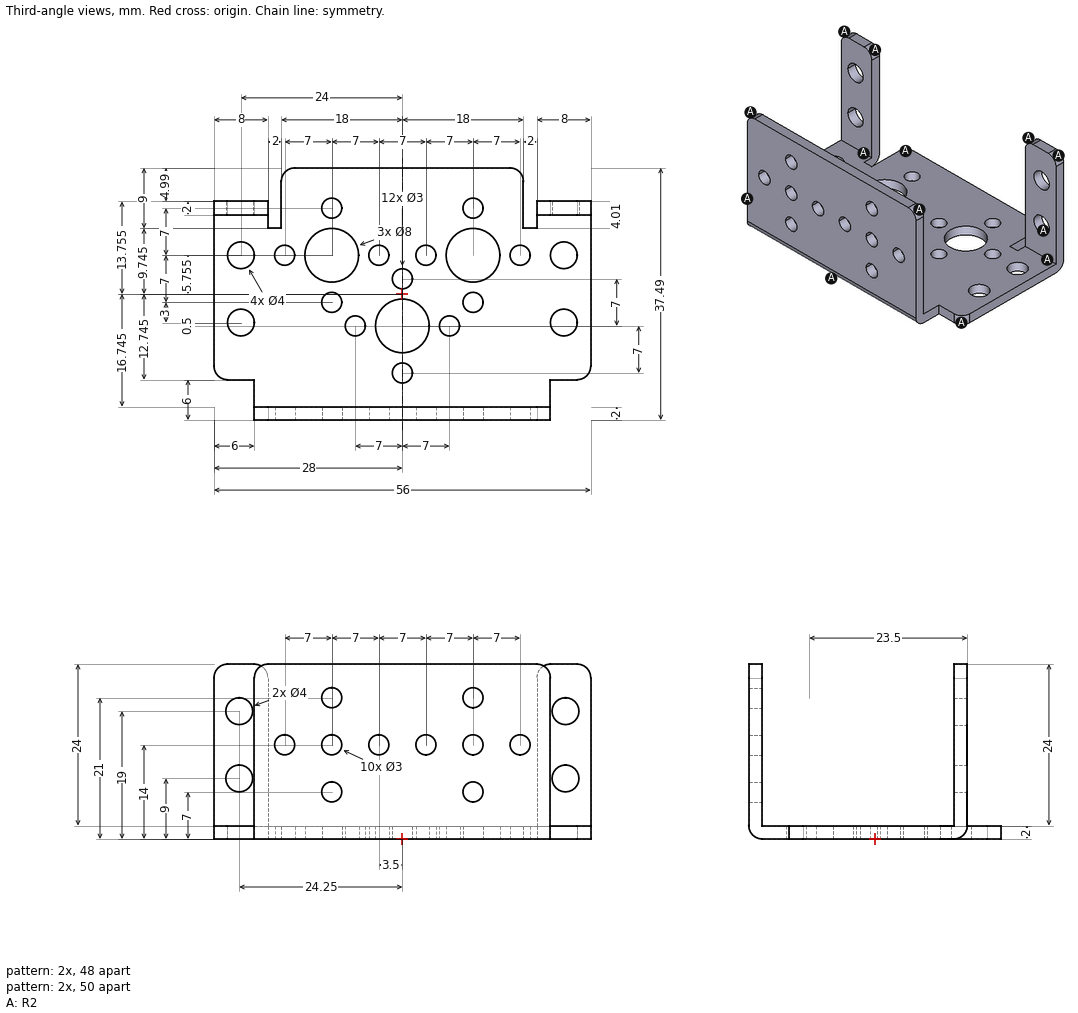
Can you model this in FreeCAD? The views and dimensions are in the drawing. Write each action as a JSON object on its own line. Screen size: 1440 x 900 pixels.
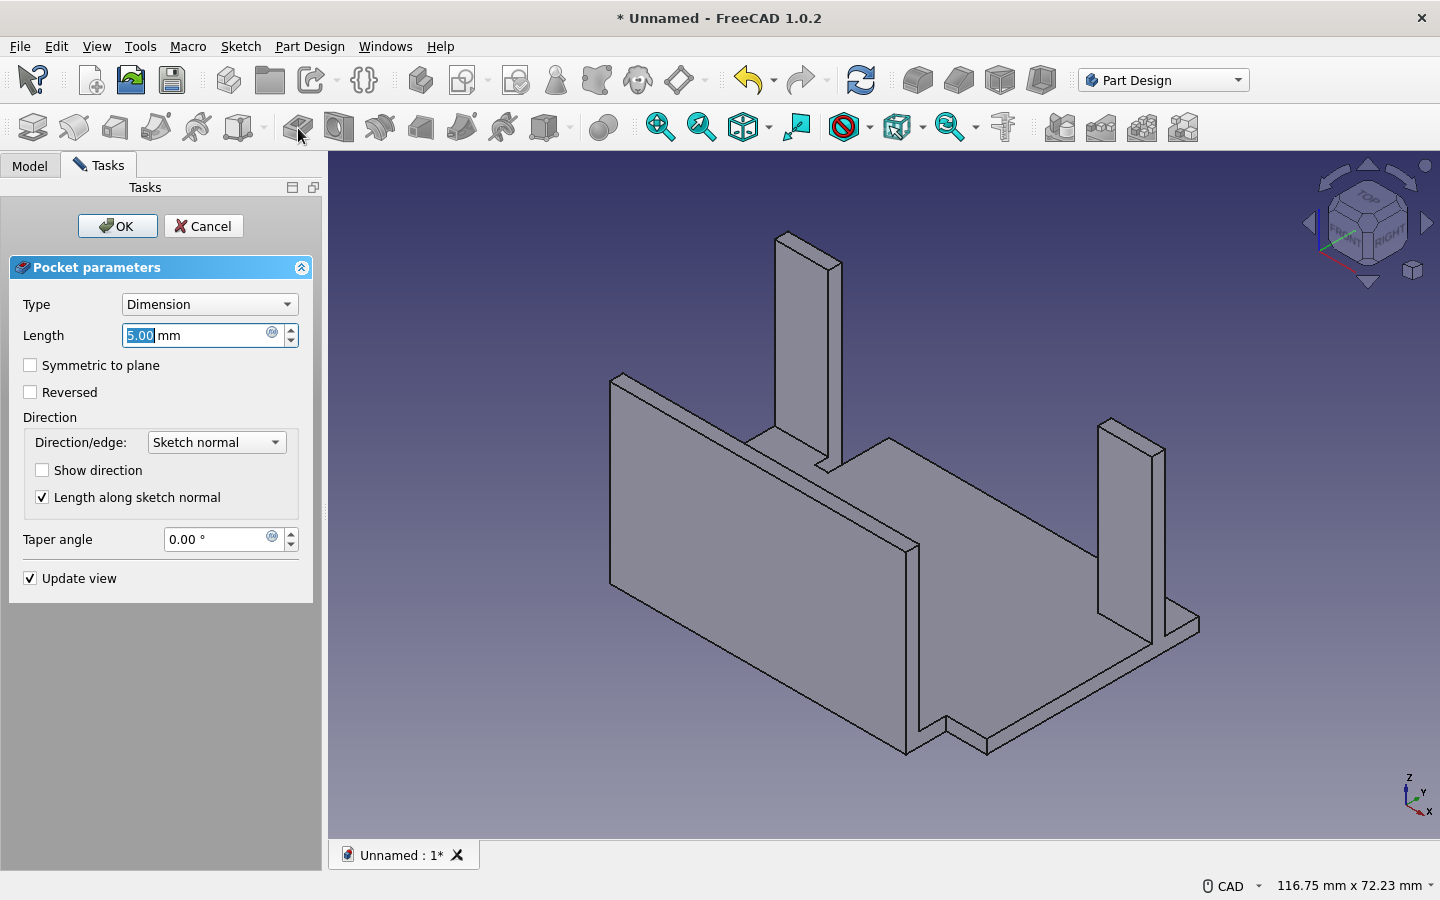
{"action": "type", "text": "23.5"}
{"action": "key", "text": "Tab"}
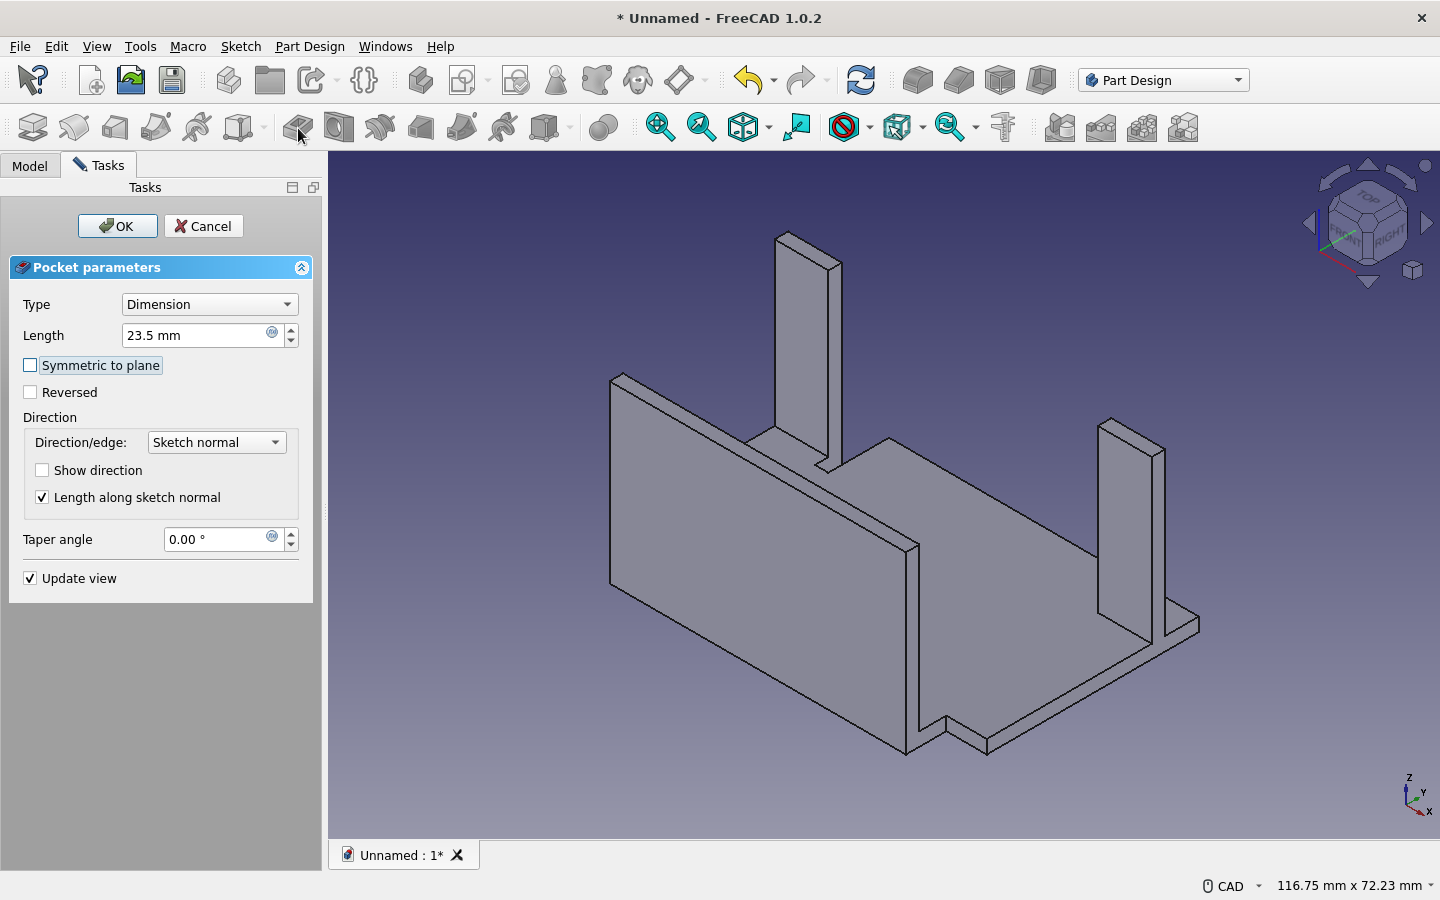
{"action": "left_click", "coordinate": [118, 226]}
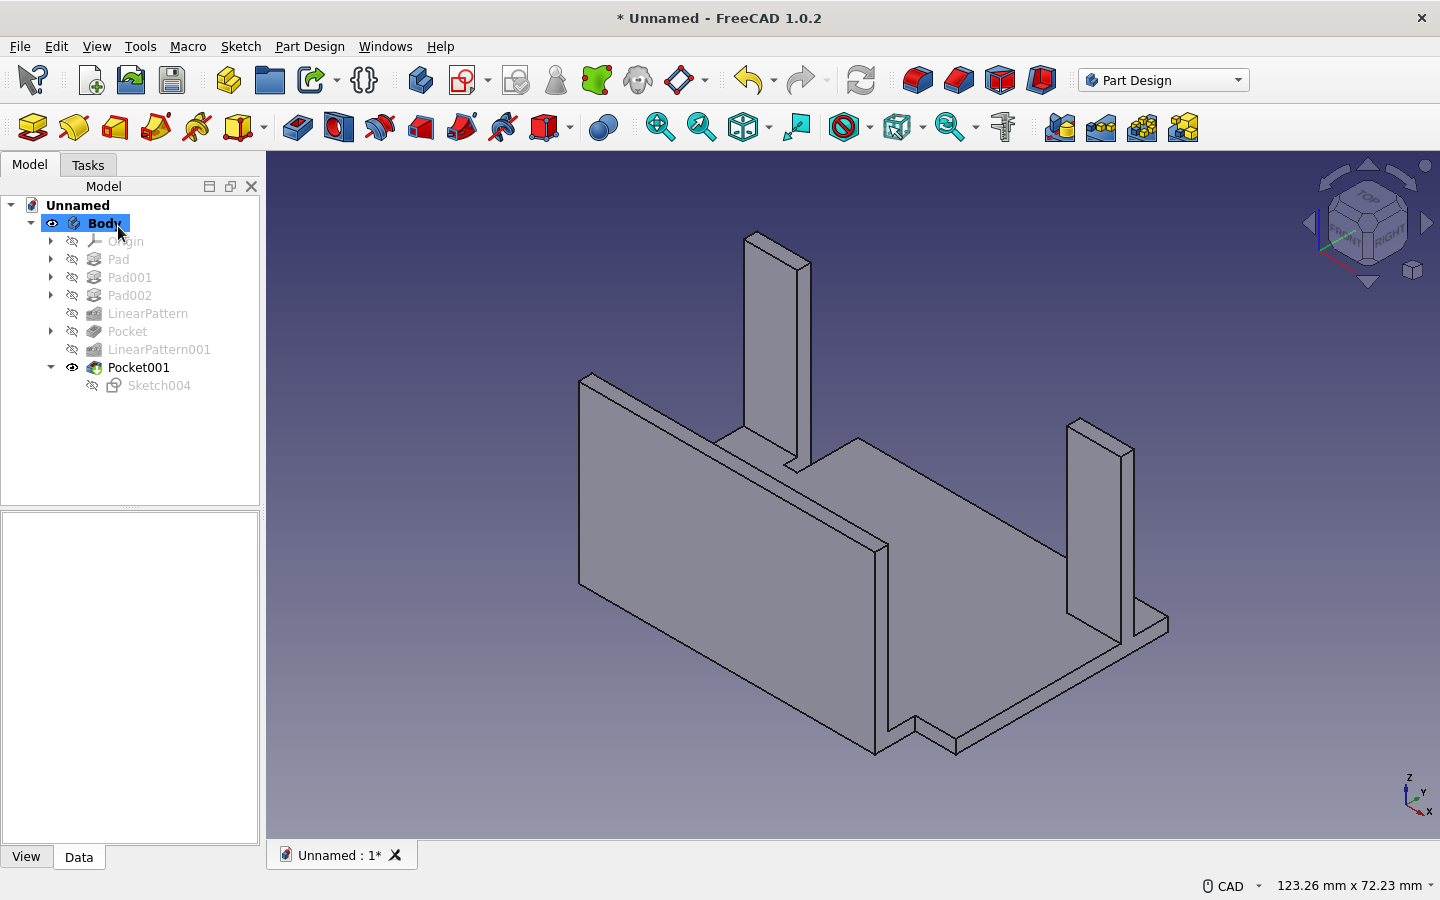
{"action": "left_click", "coordinate": [914, 607]}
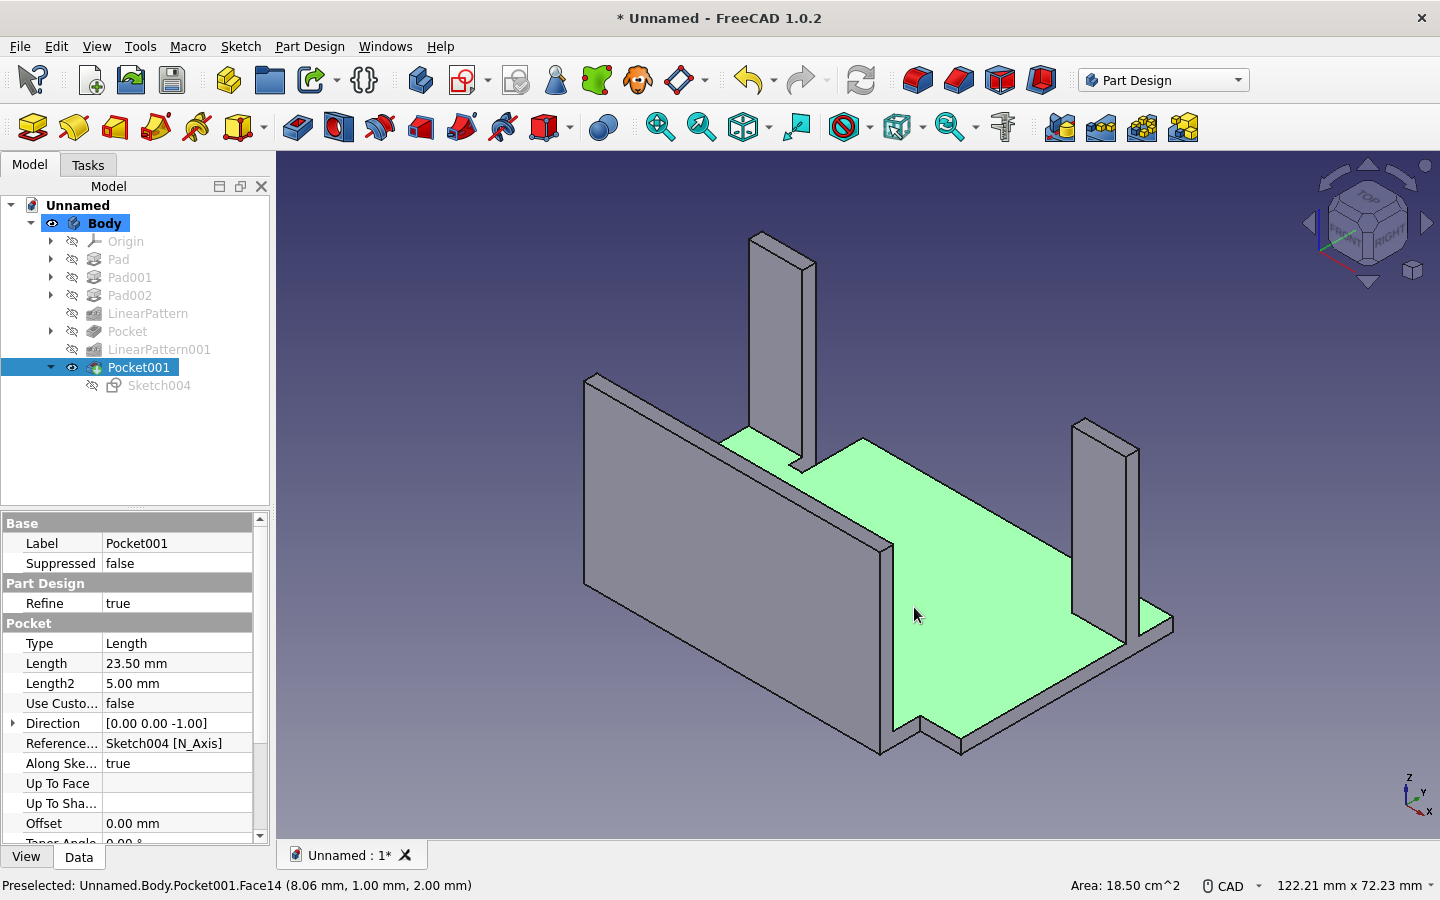
{"action": "left_click", "coordinate": [462, 80]}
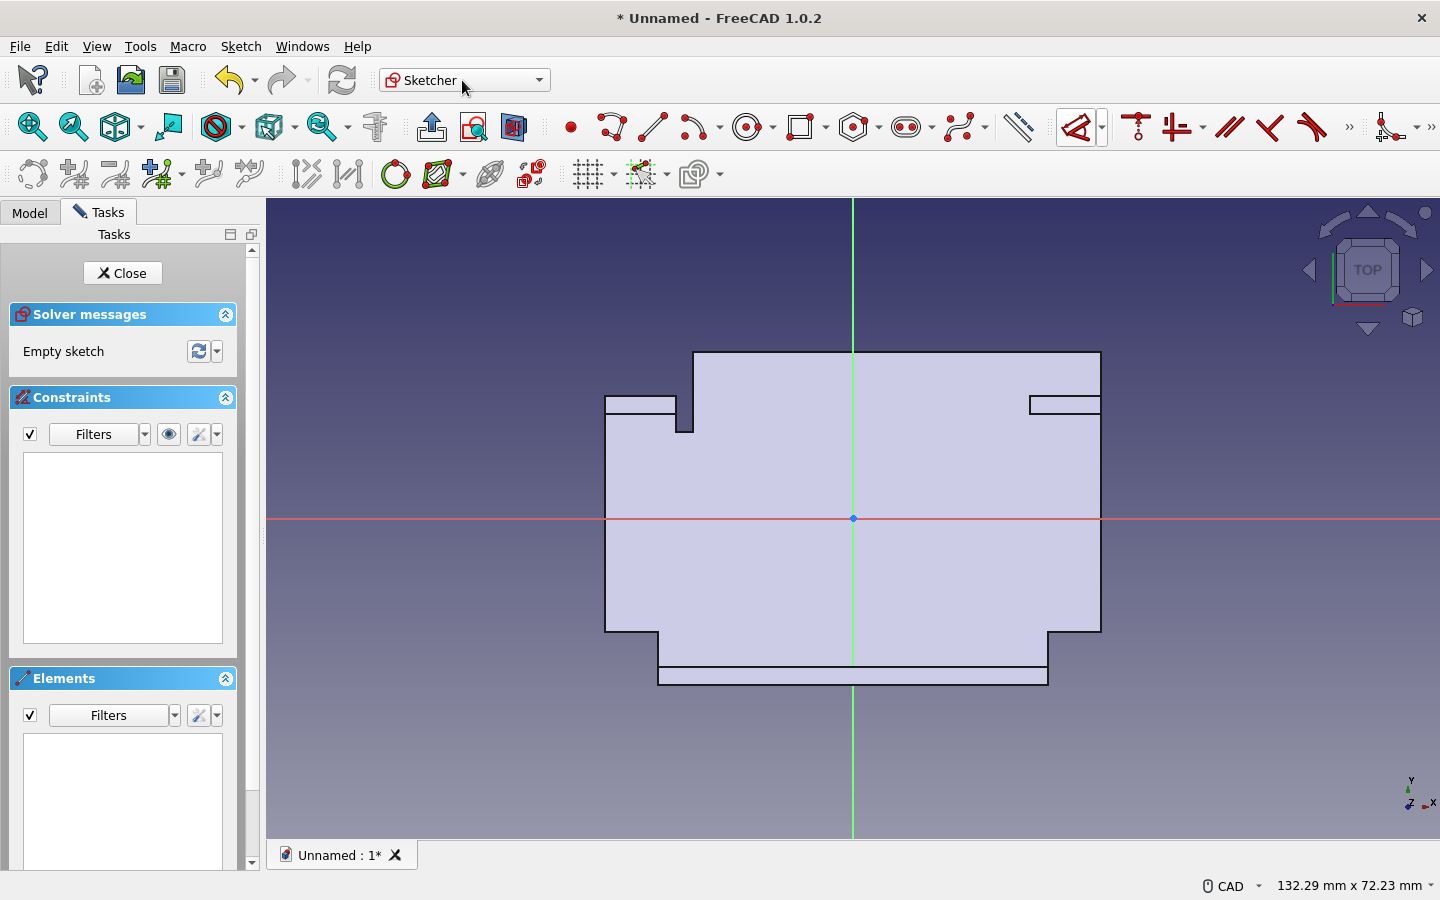
{"action": "left_click", "coordinate": [514, 128]}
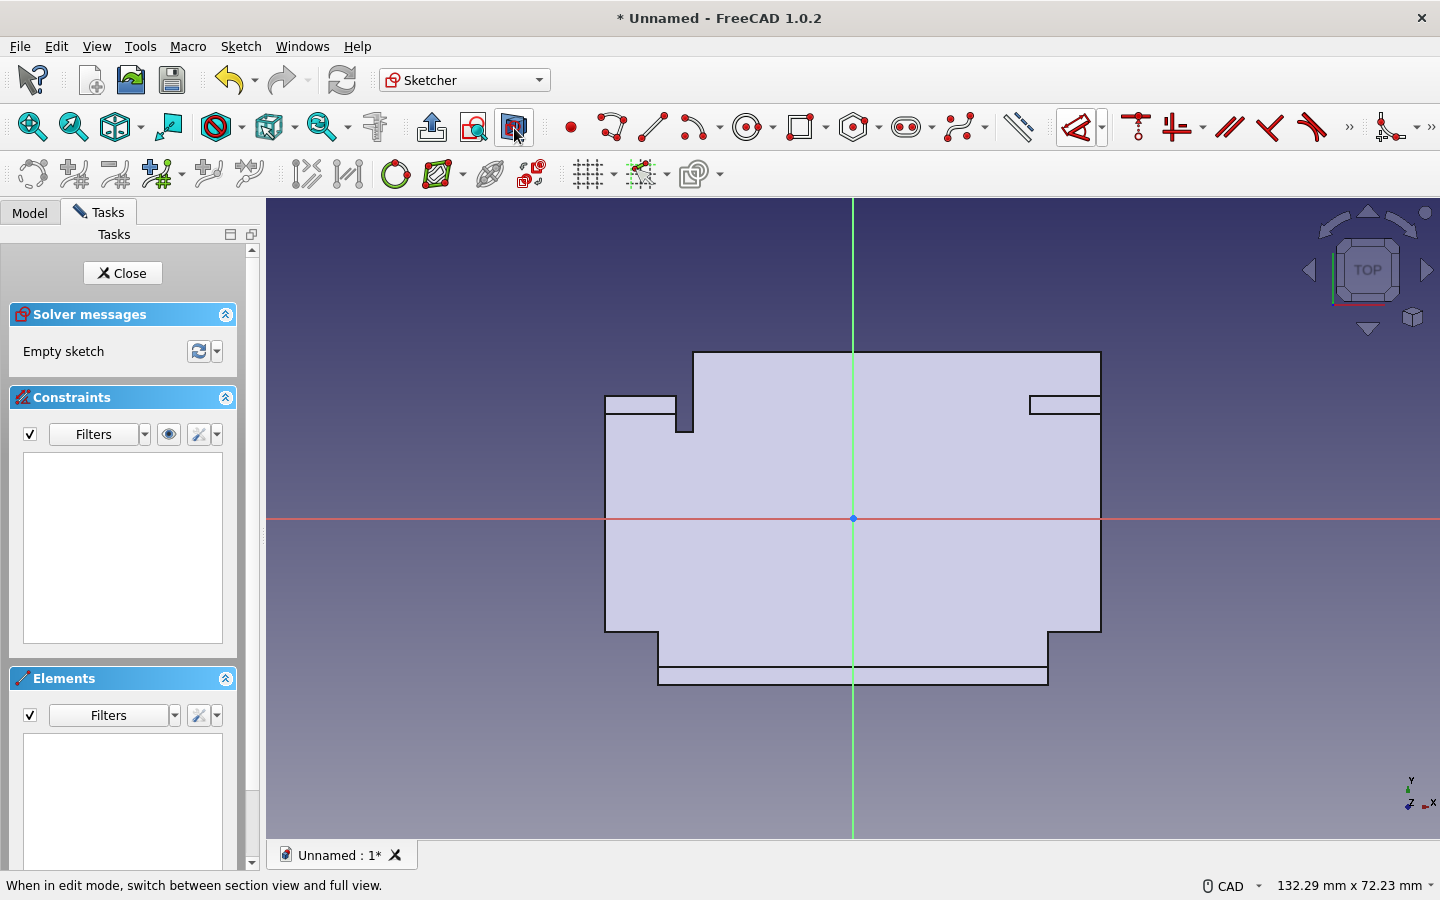
{"action": "scroll", "coordinate": [1126, 360], "scroll_direction": "up", "scroll_amount": 8}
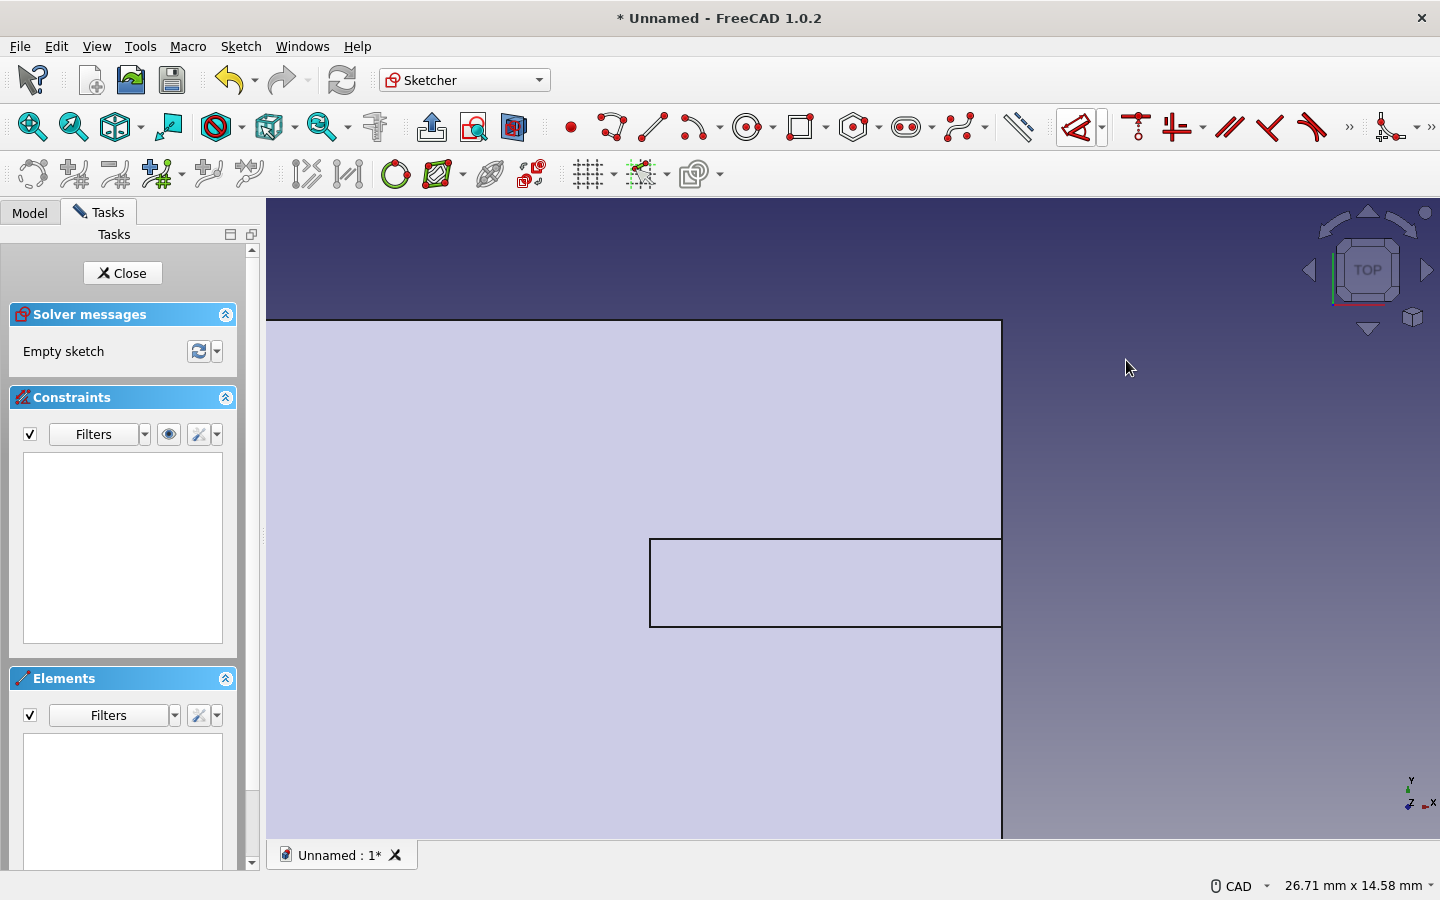
{"action": "key", "text": "g m"}